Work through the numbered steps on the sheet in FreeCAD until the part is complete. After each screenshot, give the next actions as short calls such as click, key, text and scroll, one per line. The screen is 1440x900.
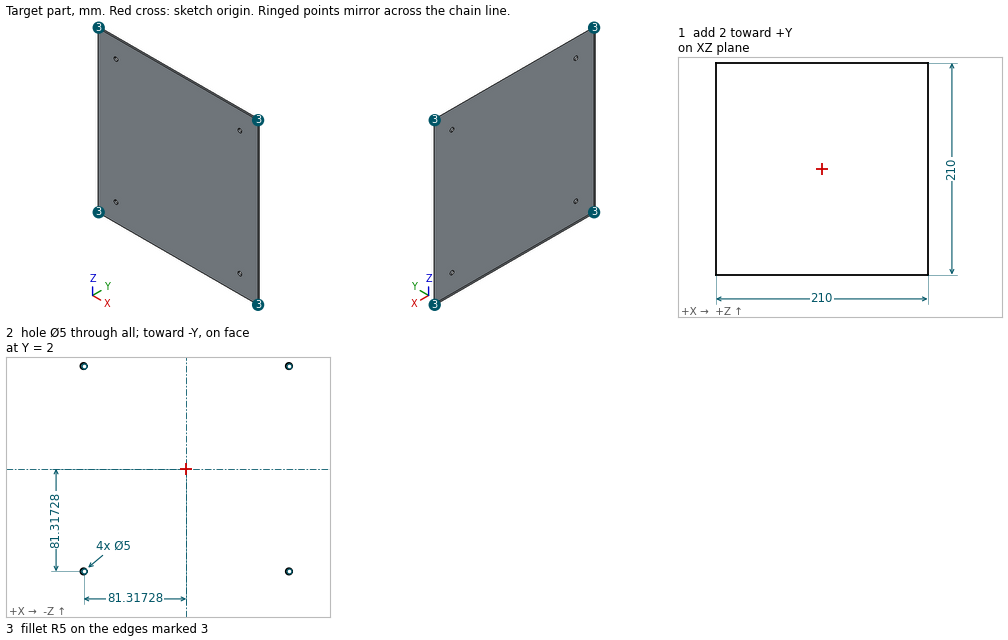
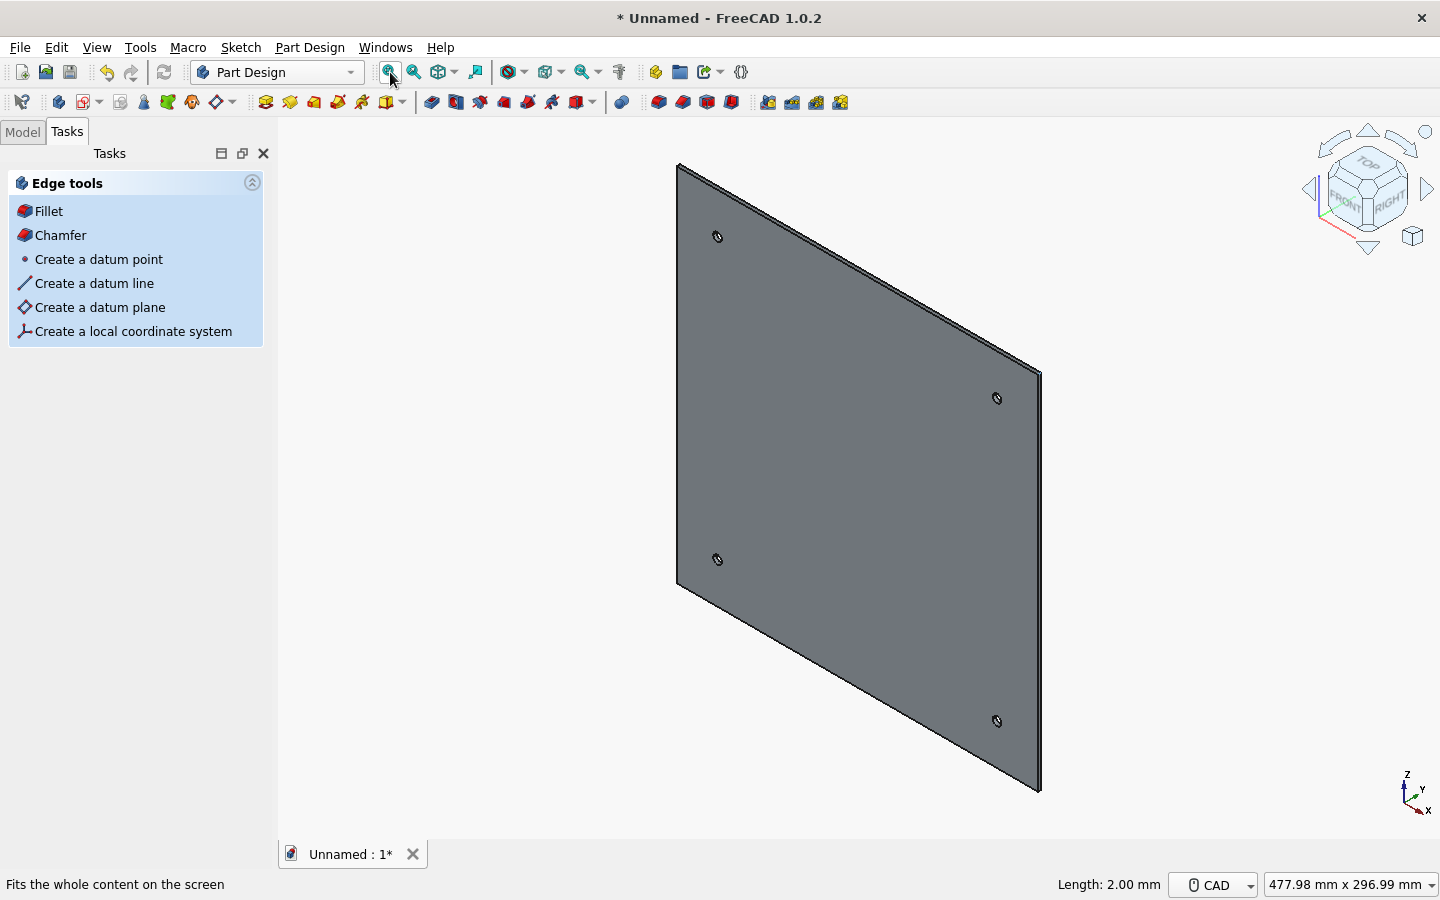
key(2)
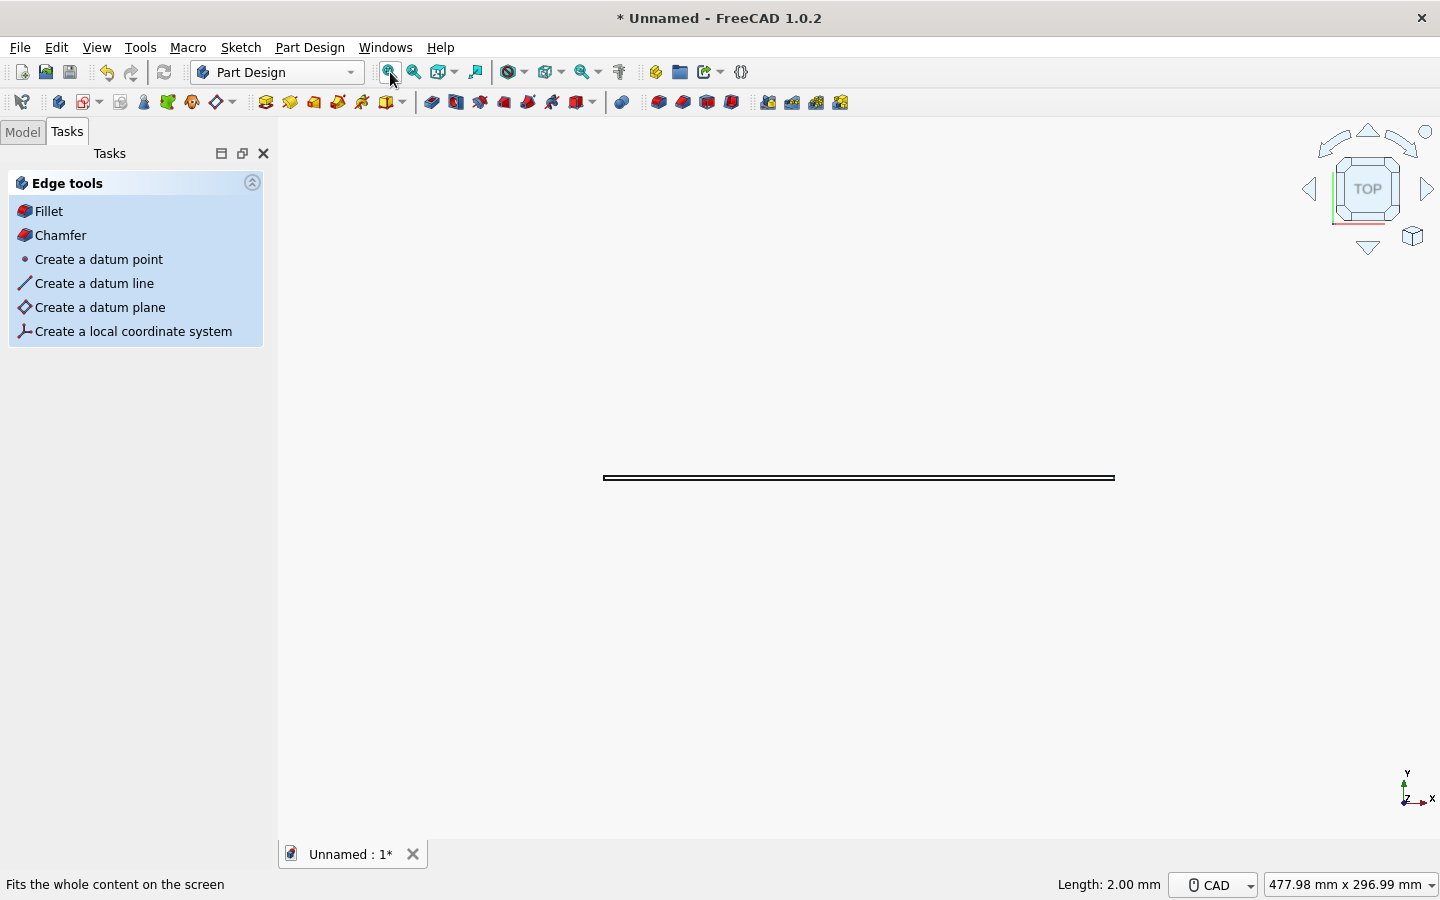
click(390, 72)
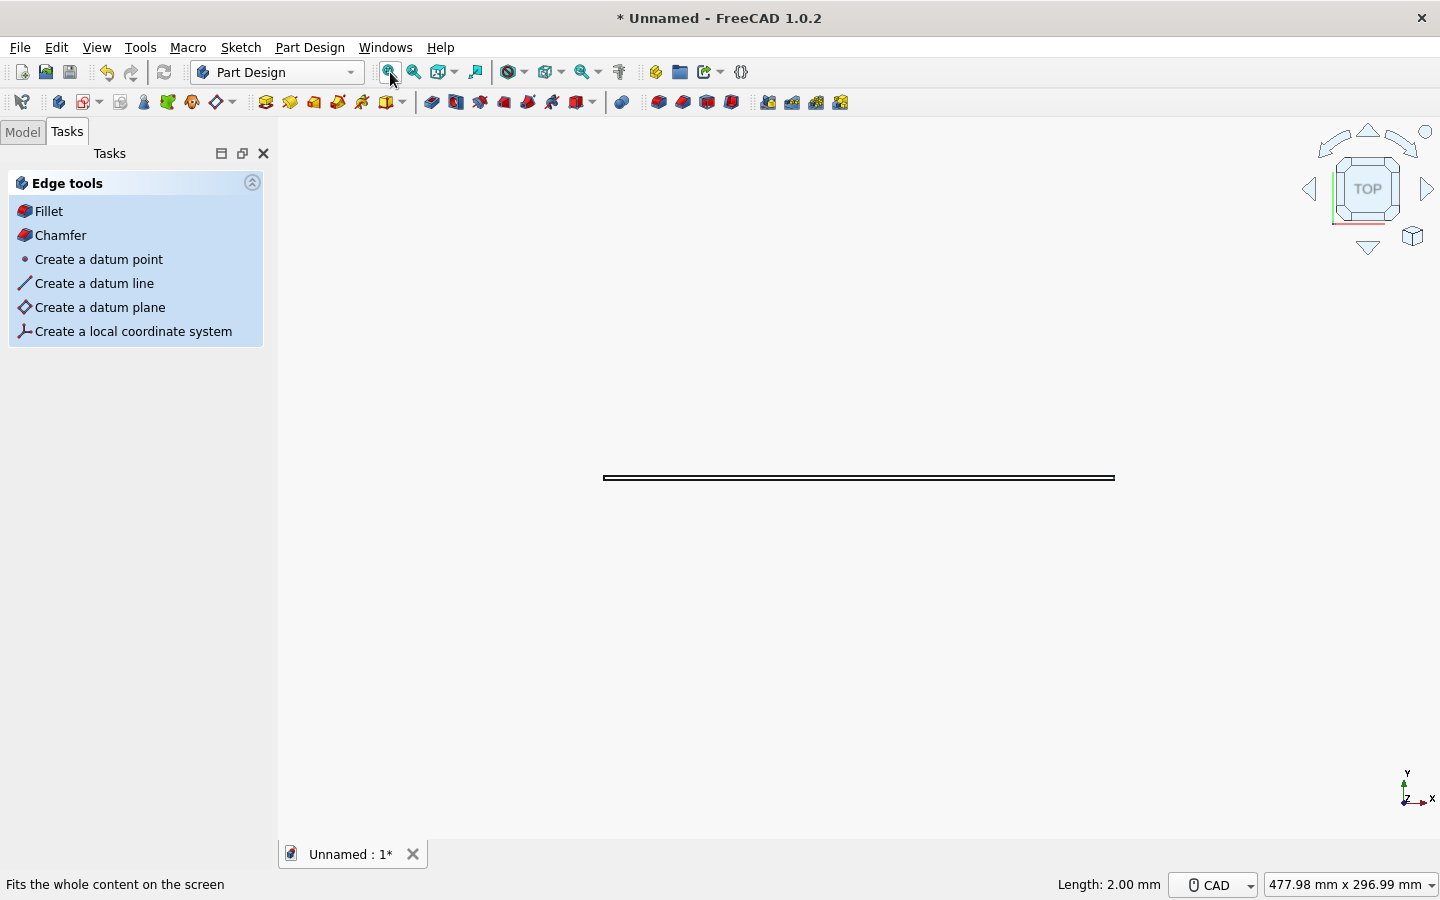
scroll(604, 477, up, 11)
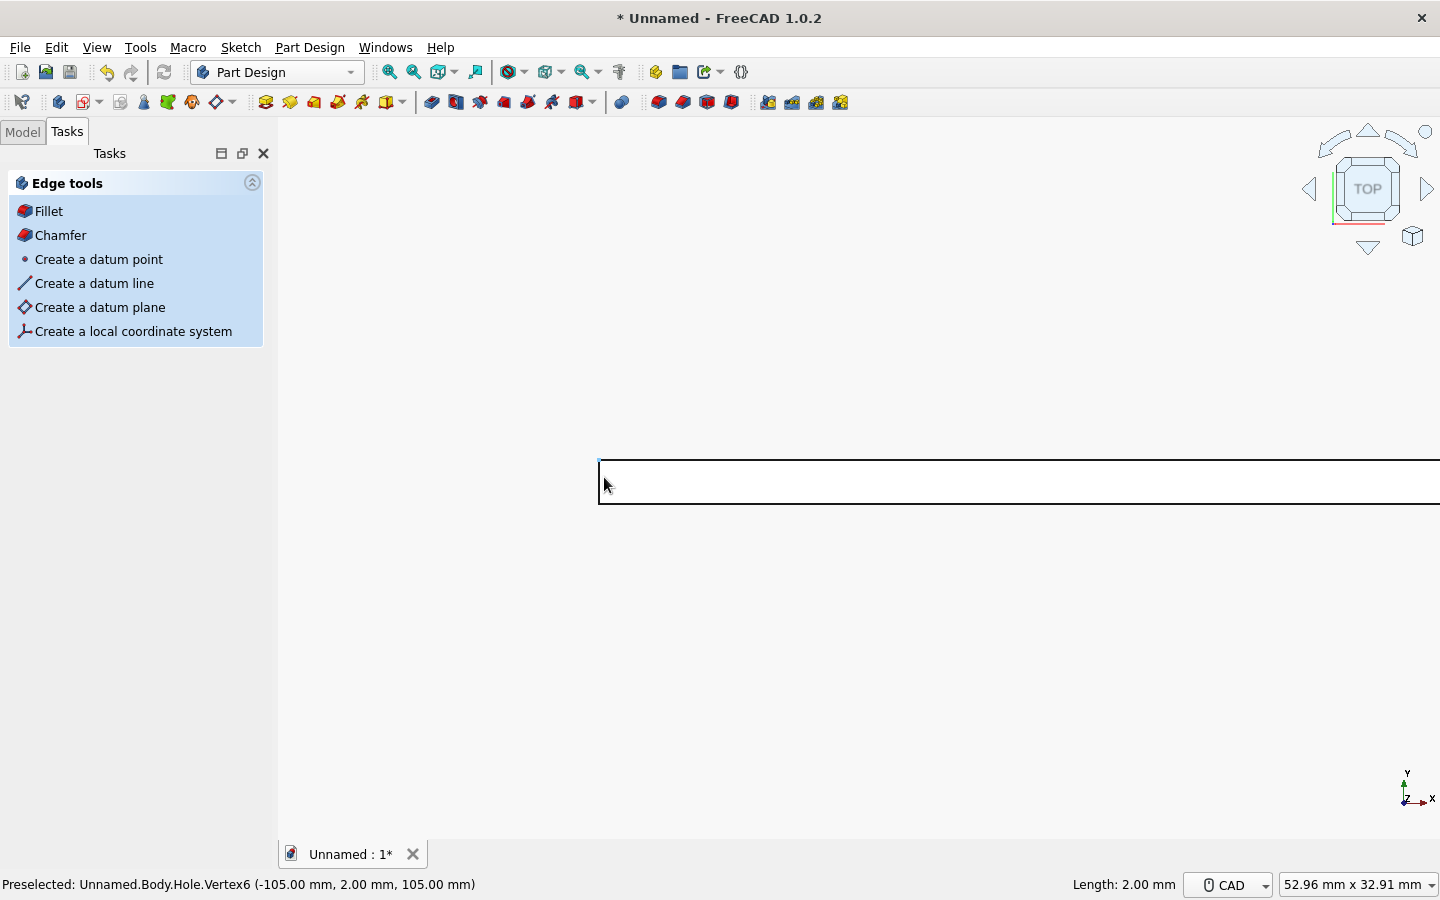
click(599, 481, ctrl)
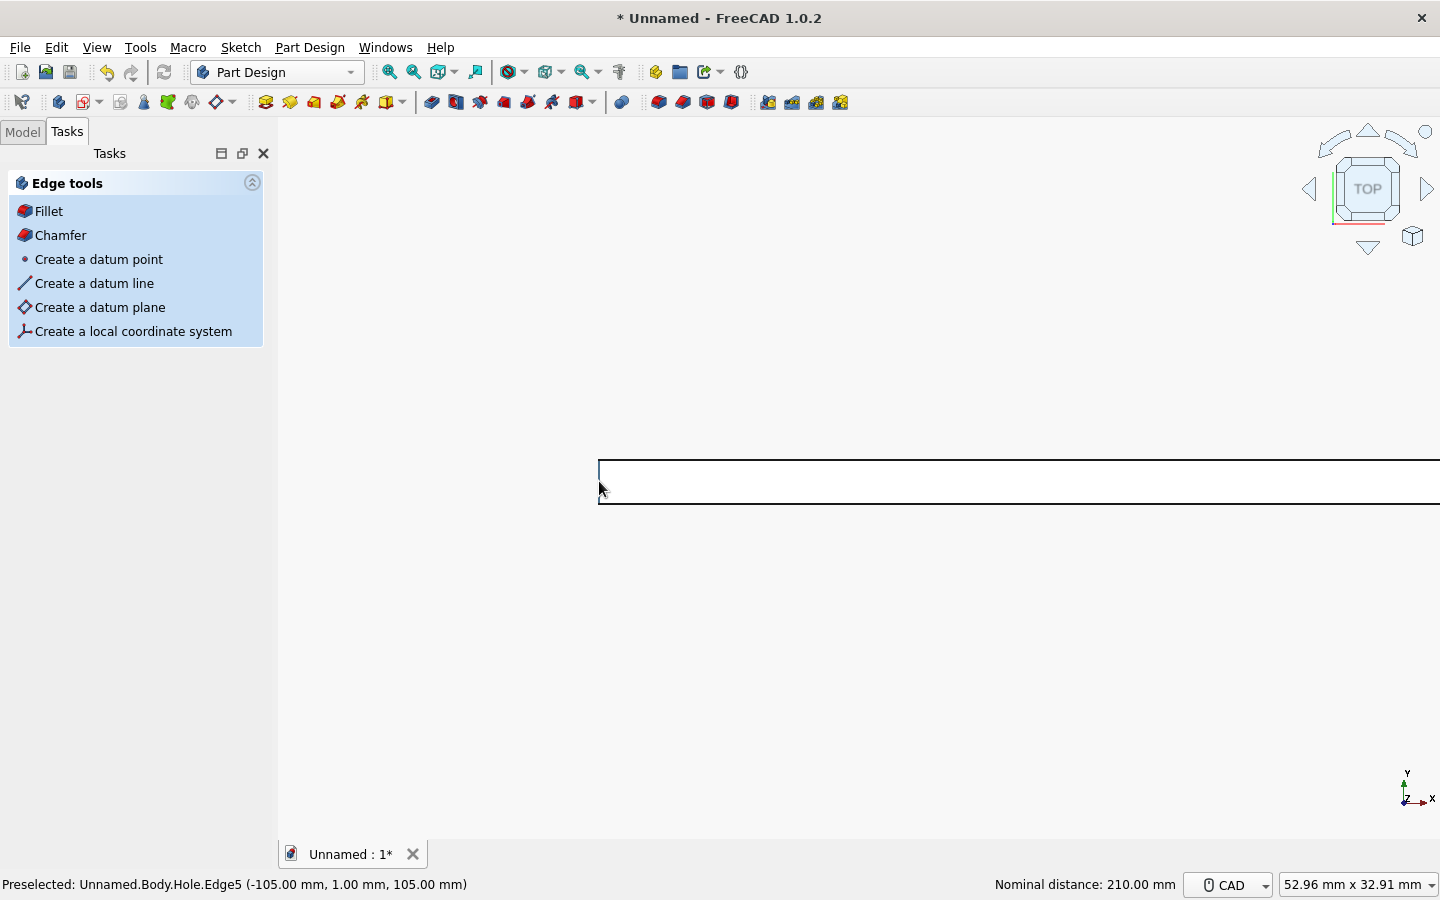
click(390, 72)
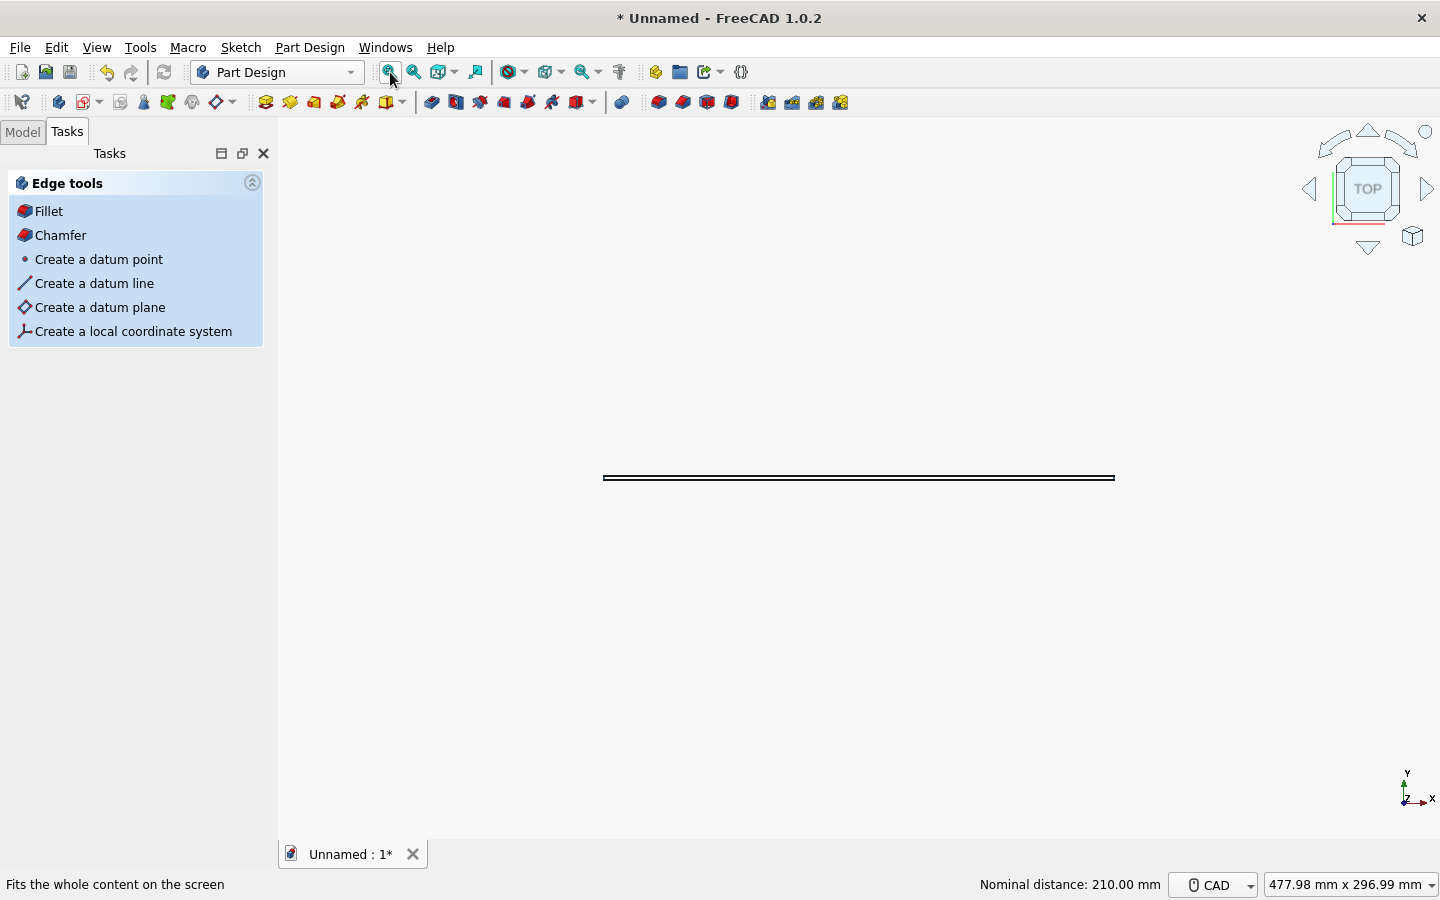
key(1)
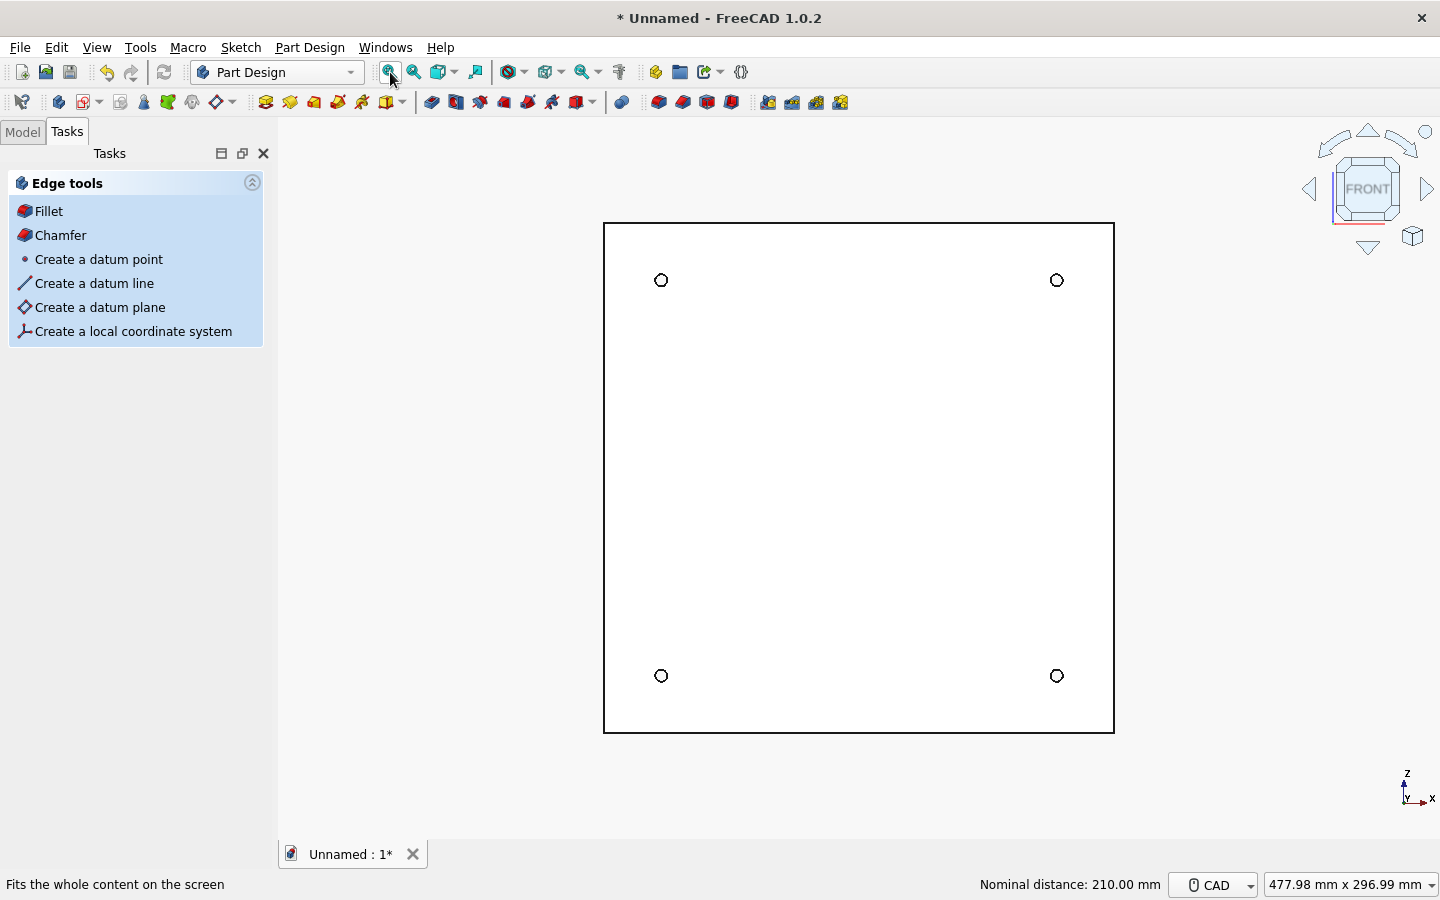
scroll(604, 732, up, 11)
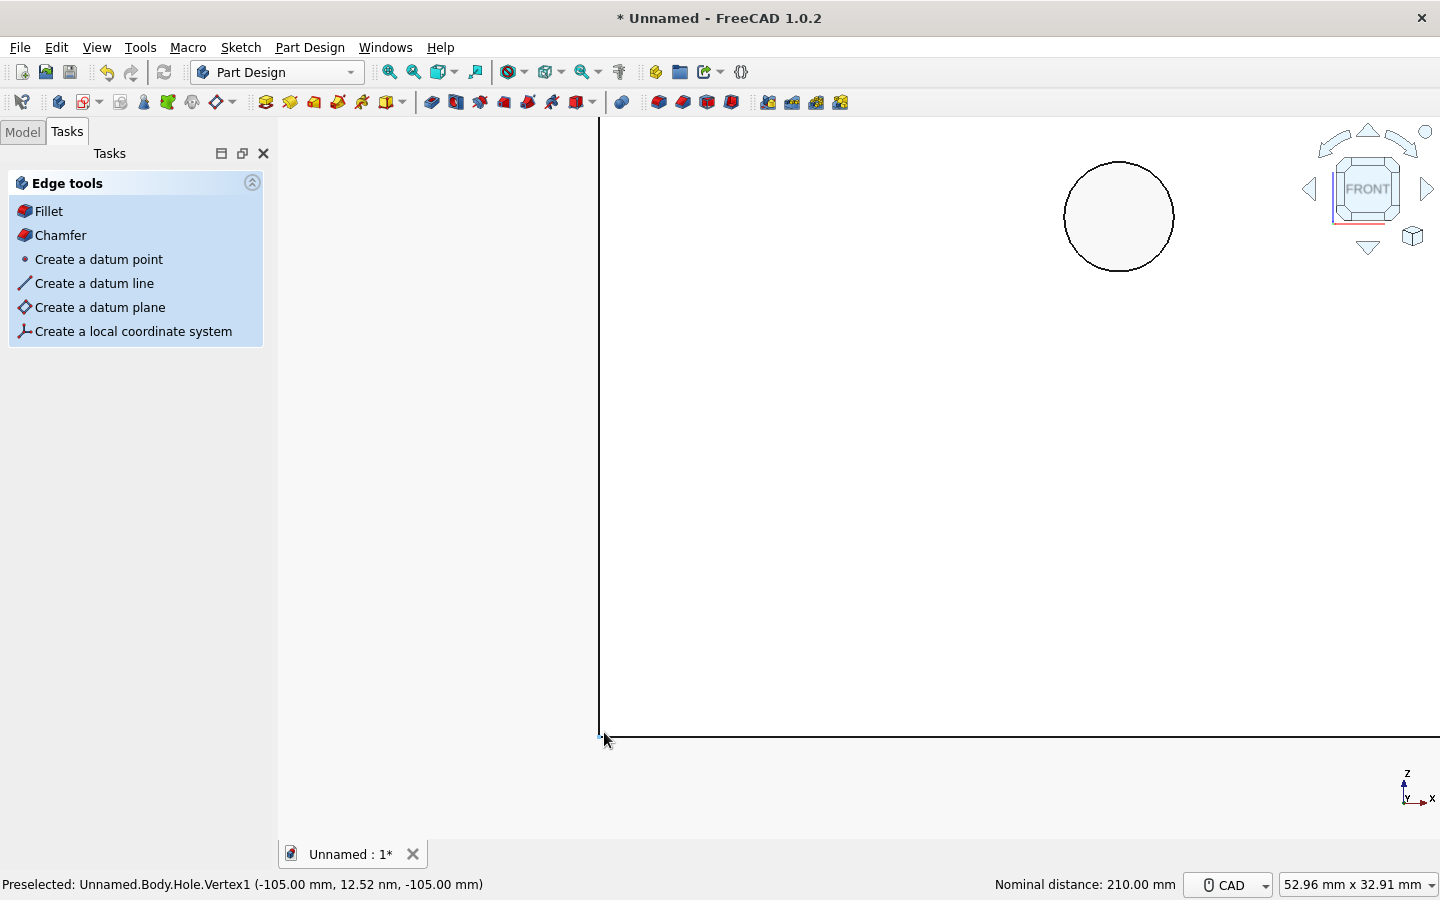
click(390, 72)